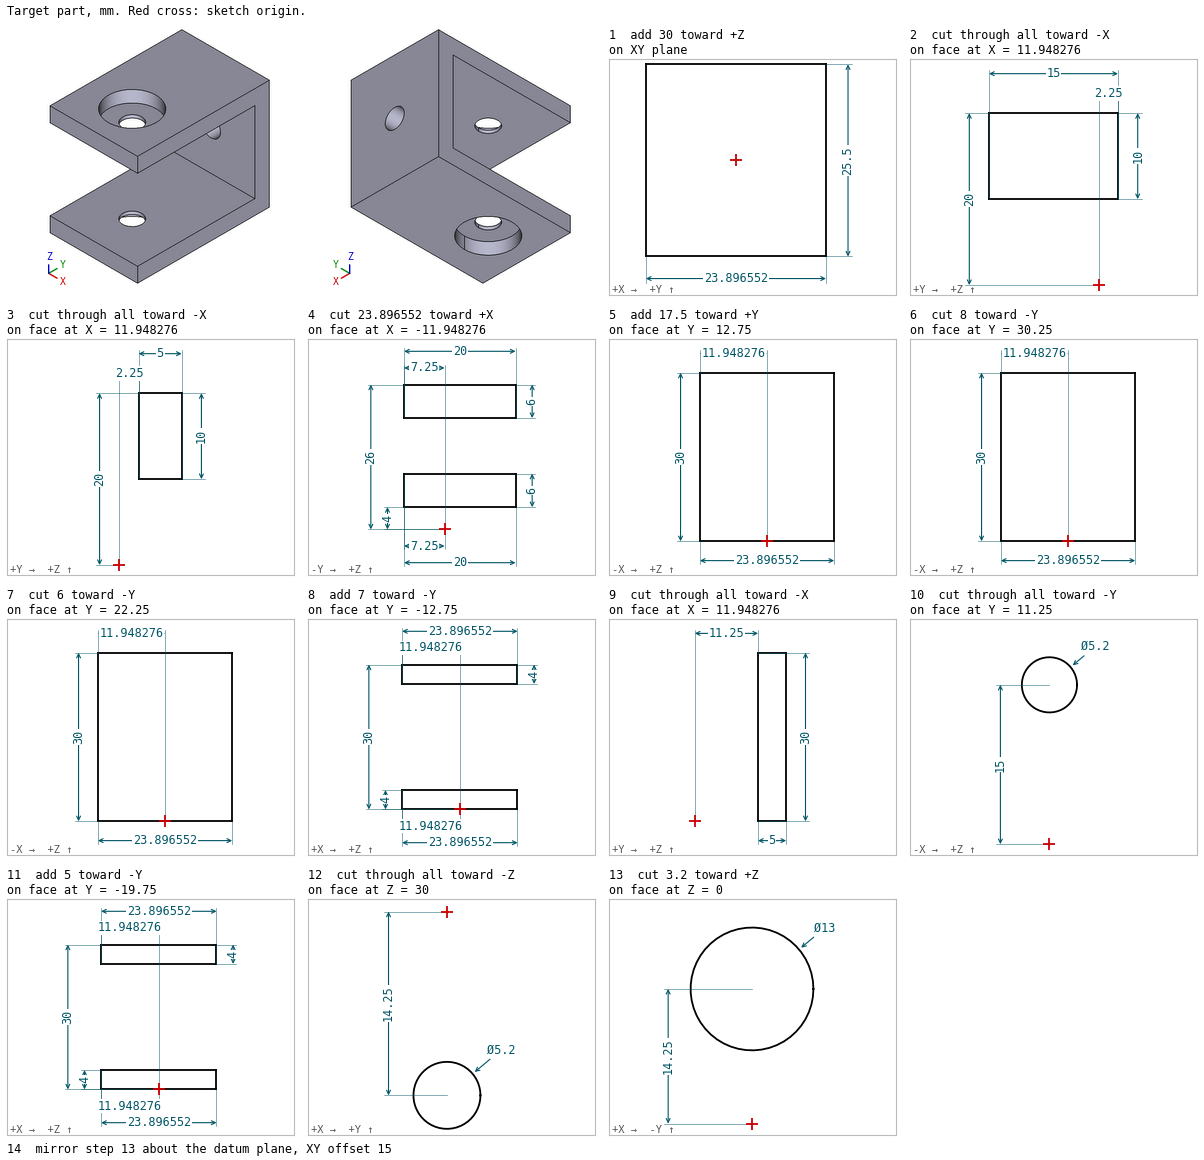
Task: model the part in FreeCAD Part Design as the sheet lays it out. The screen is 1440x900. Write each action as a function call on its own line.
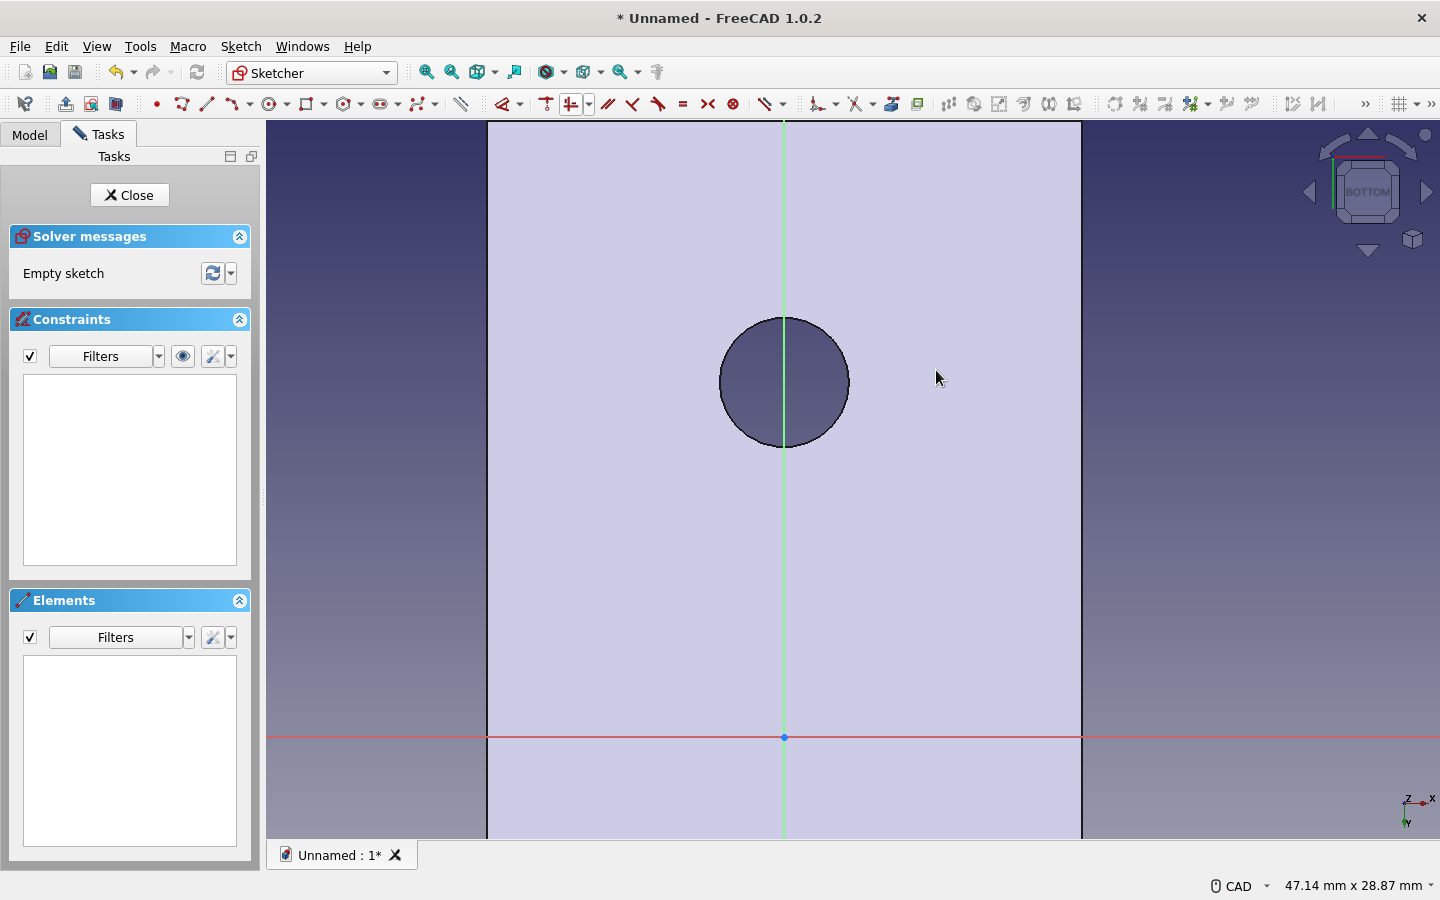
key(g)
key(c)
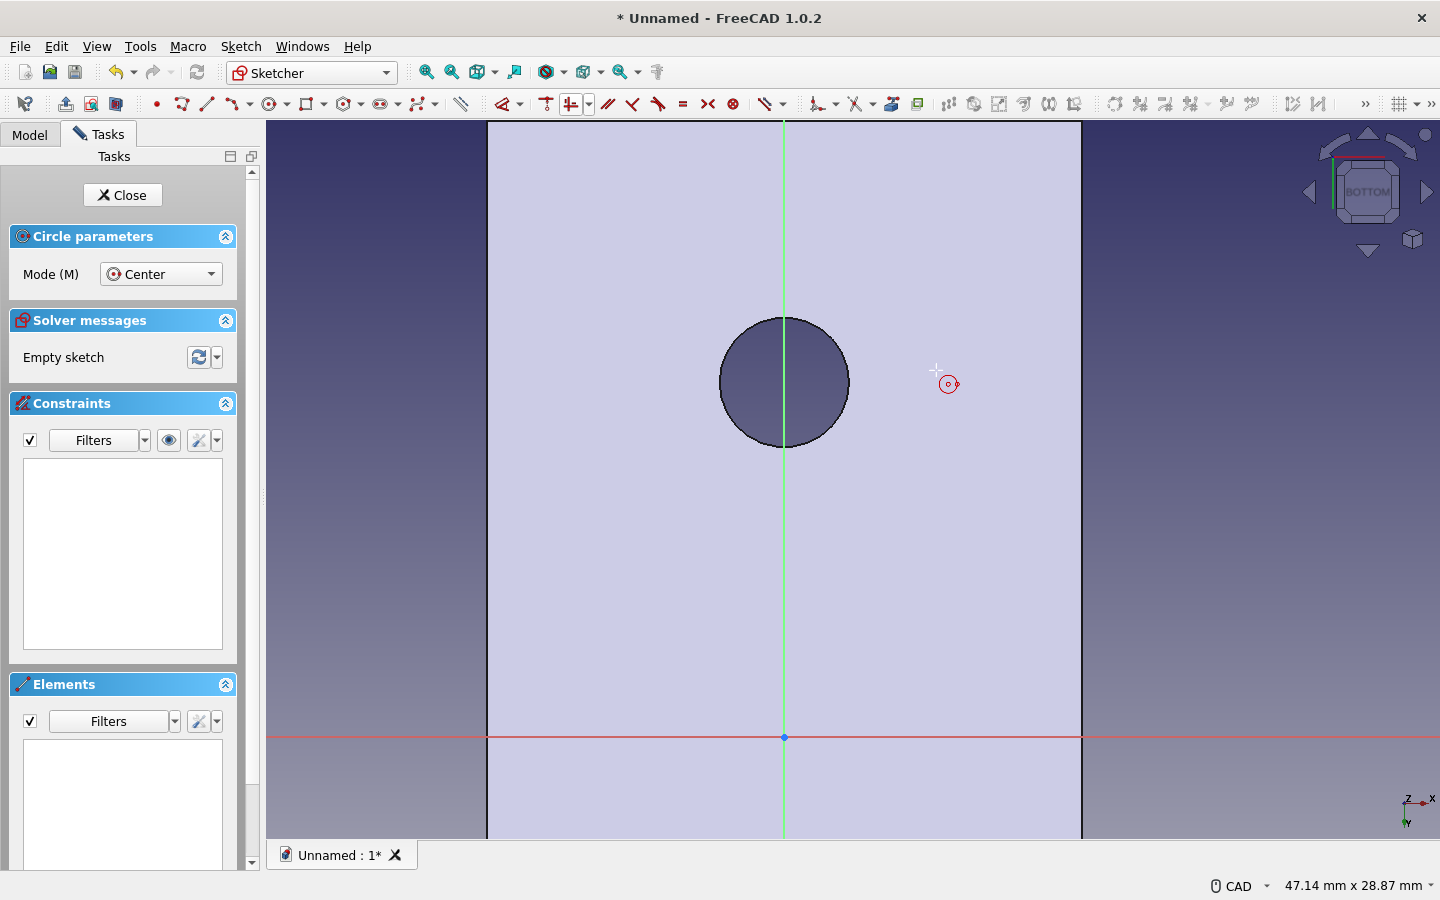
click(784, 382)
move(899, 268)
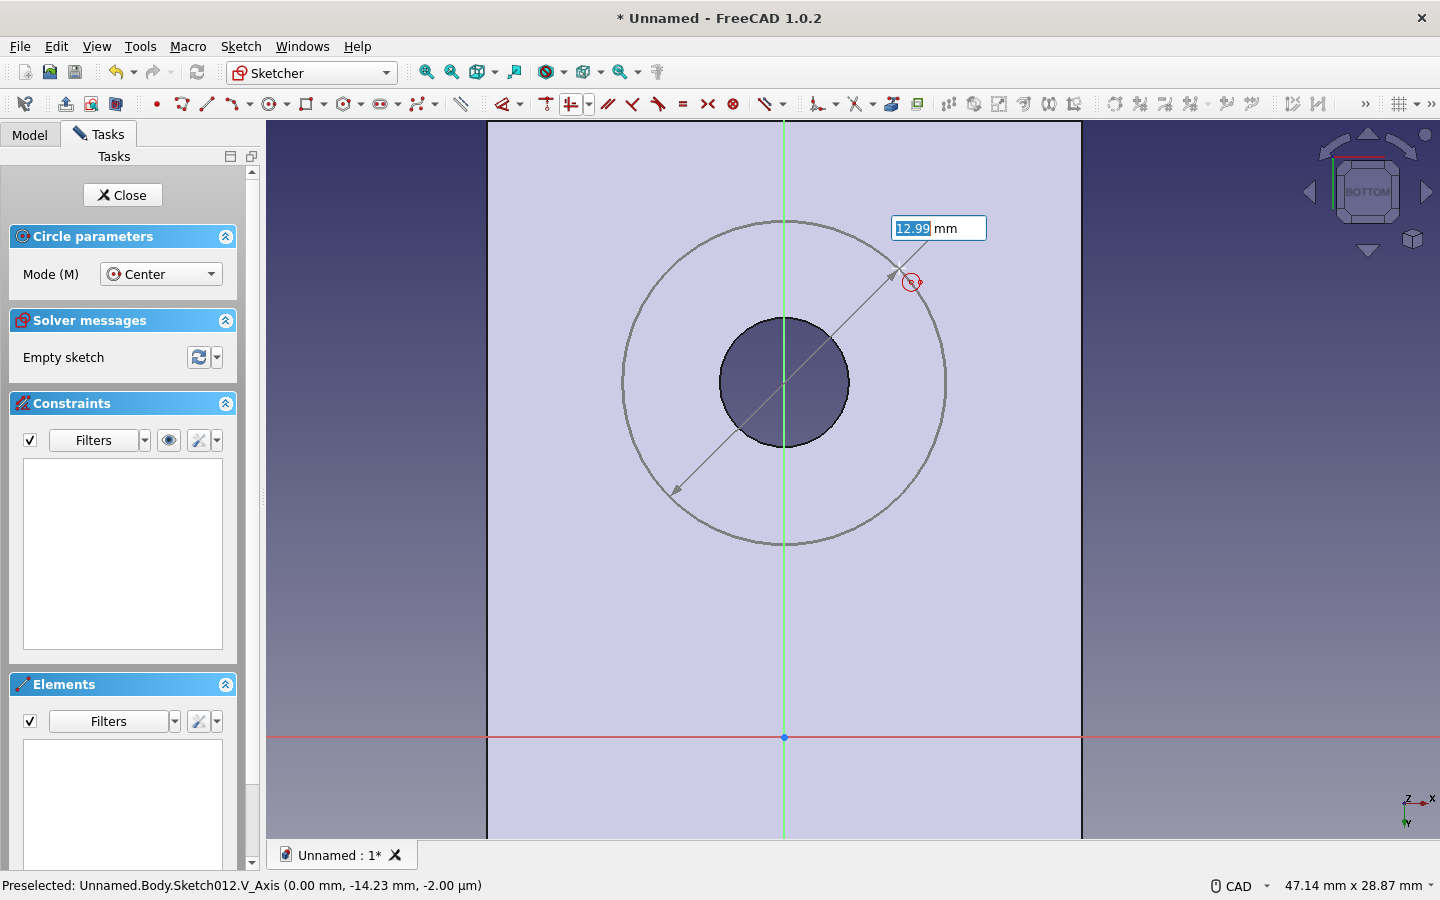
text(13)
key(Return)
key(Escape)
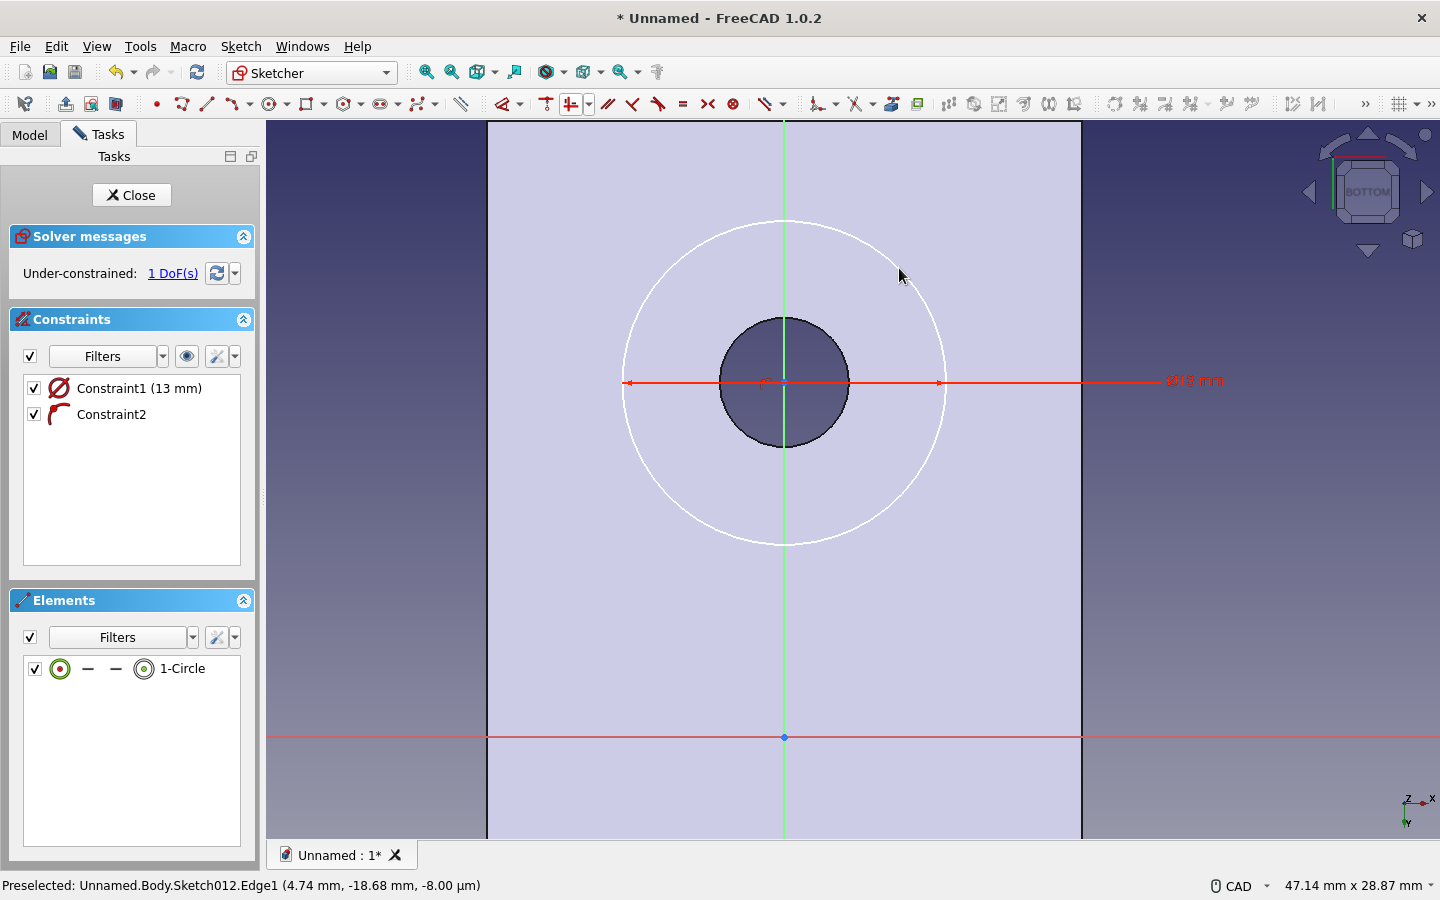
key(d)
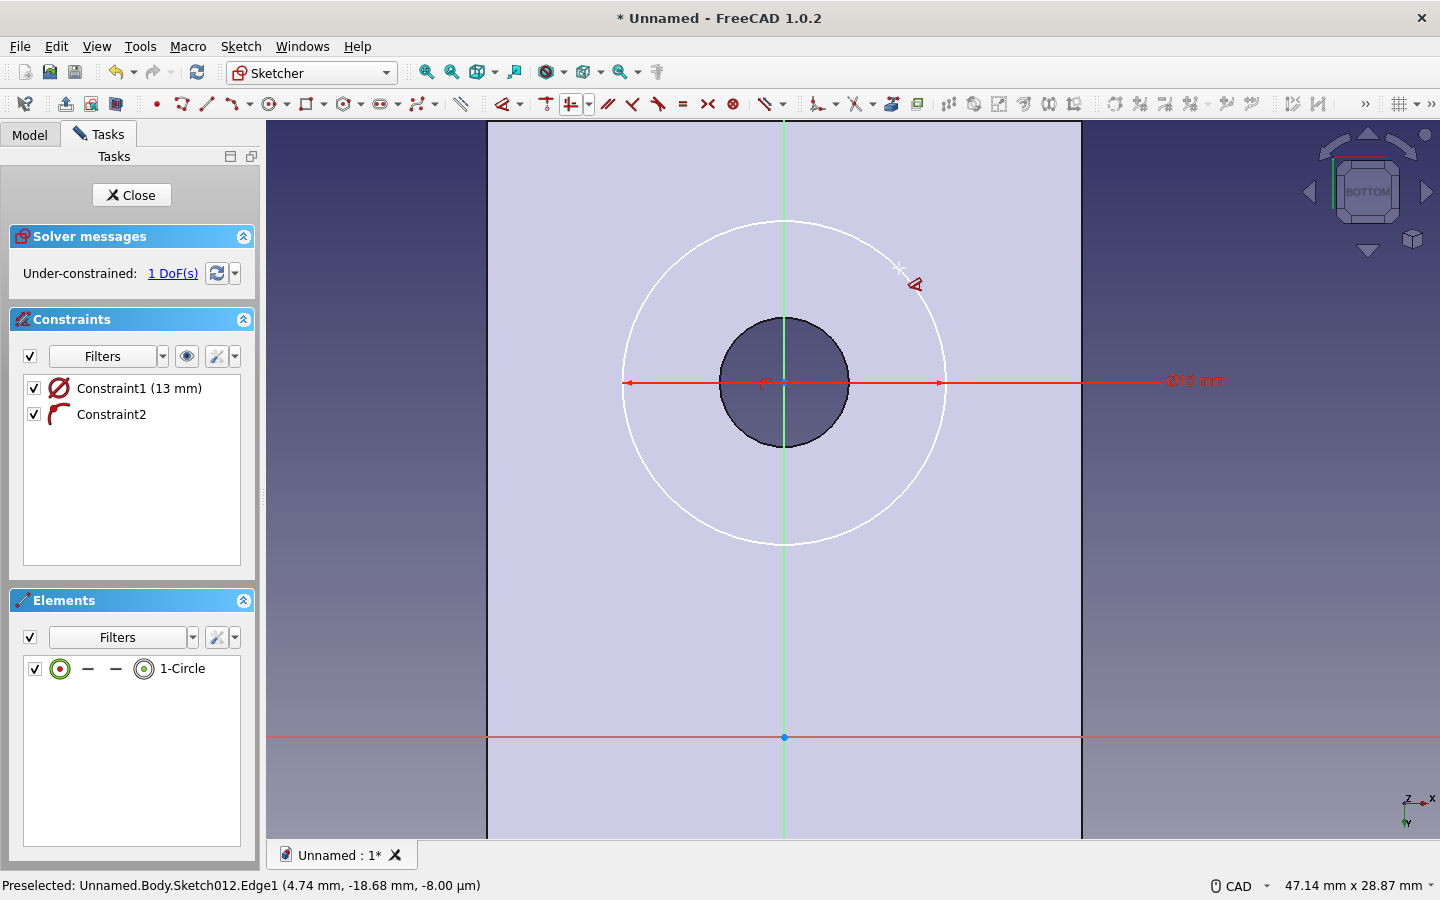
click(784, 383)
click(818, 560)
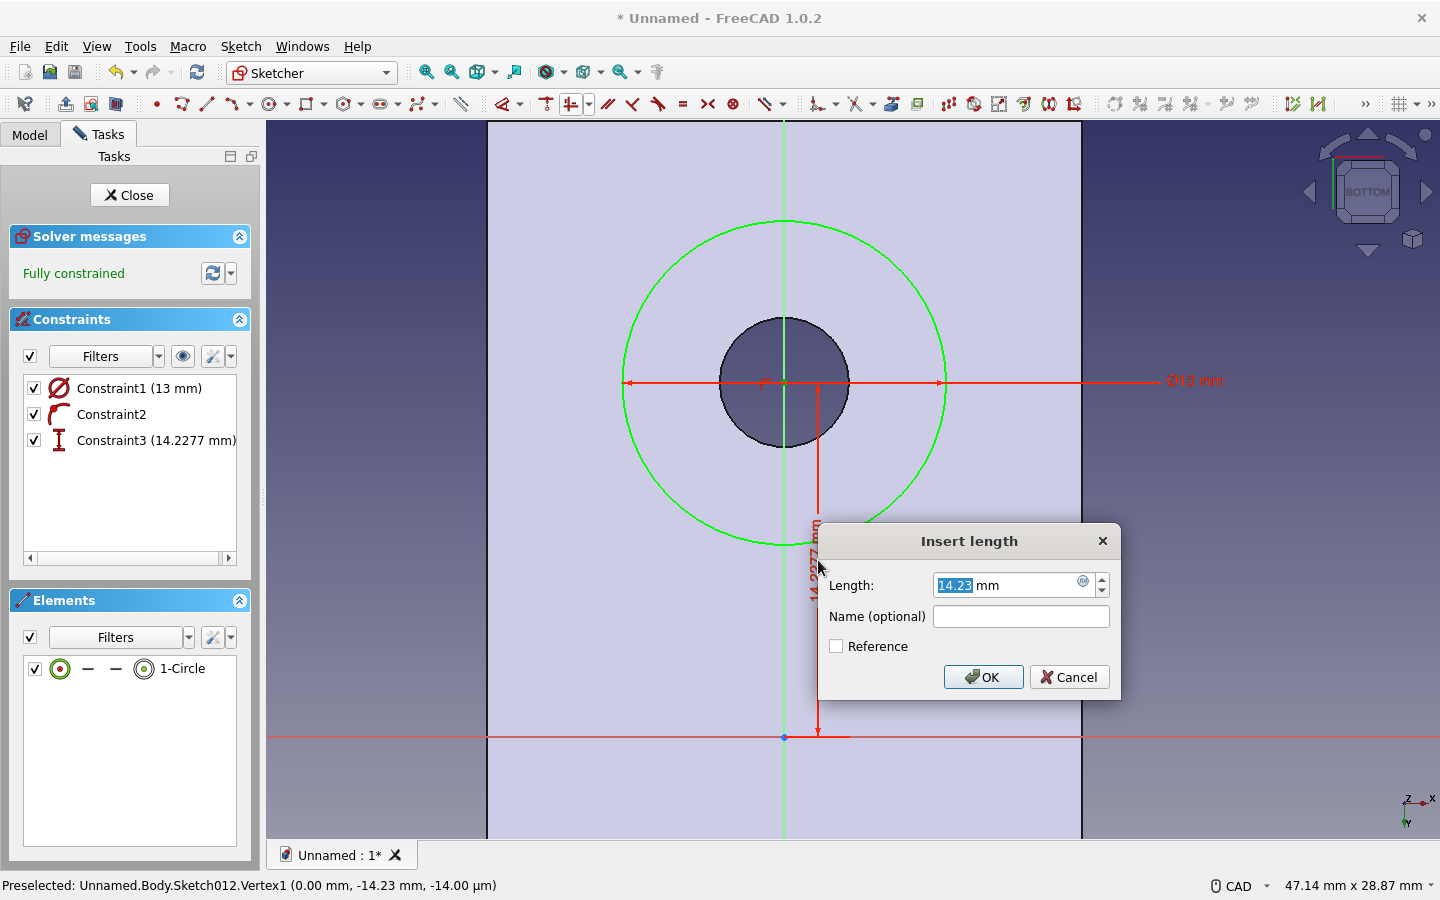
text(14.25)
key(Return)
key(Escape)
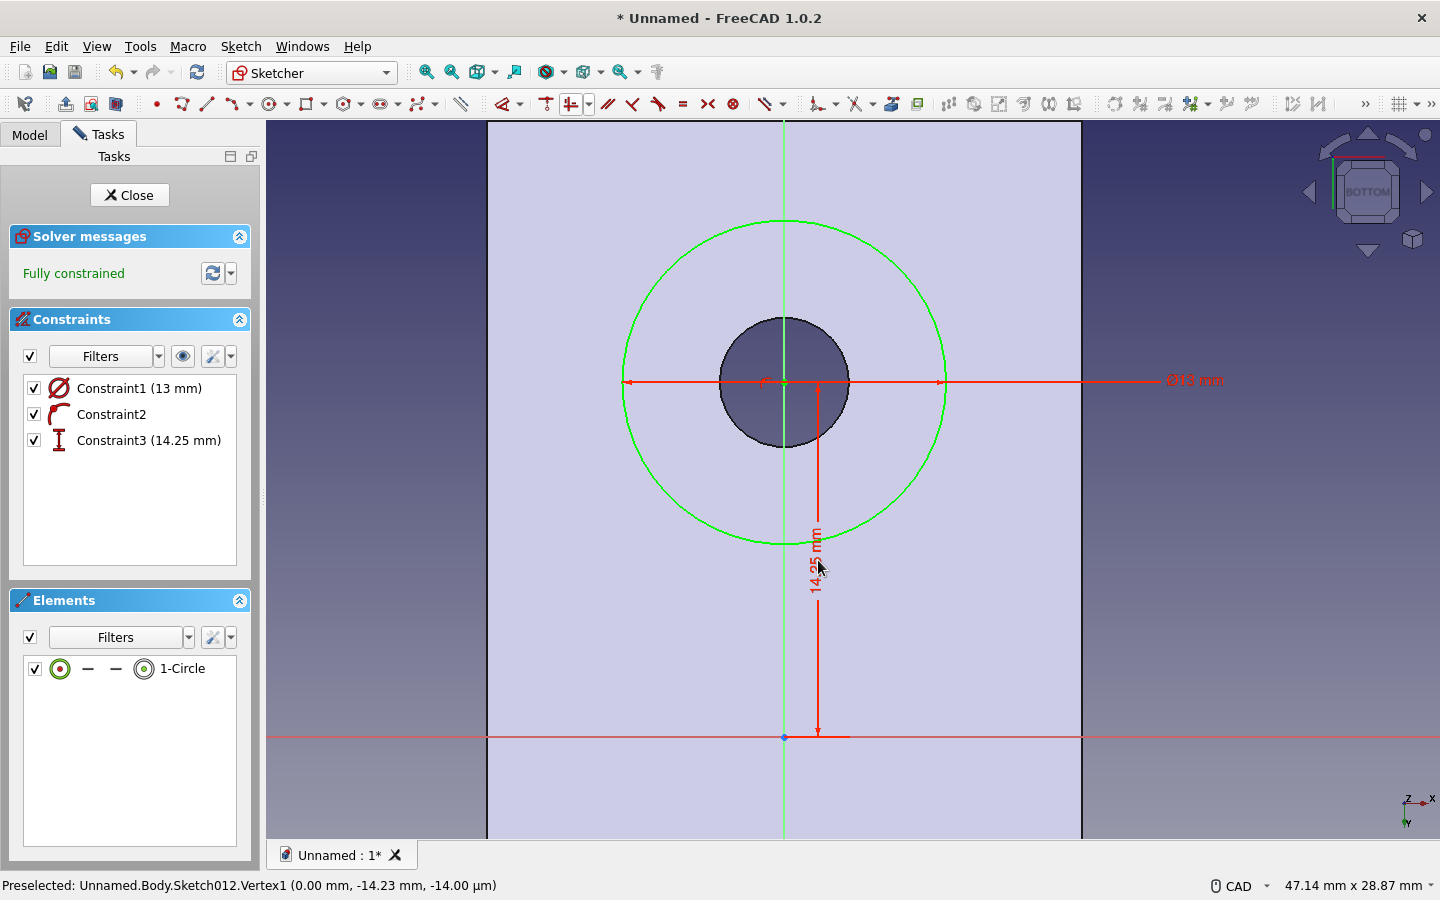
click(130, 195)